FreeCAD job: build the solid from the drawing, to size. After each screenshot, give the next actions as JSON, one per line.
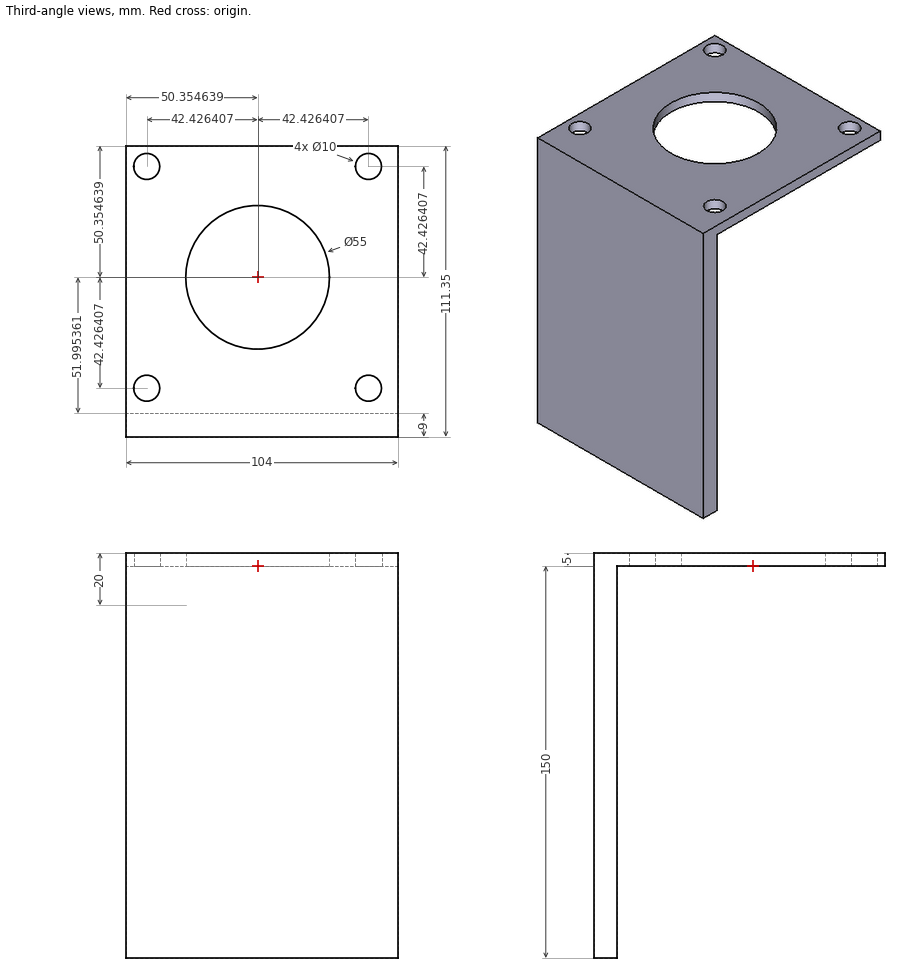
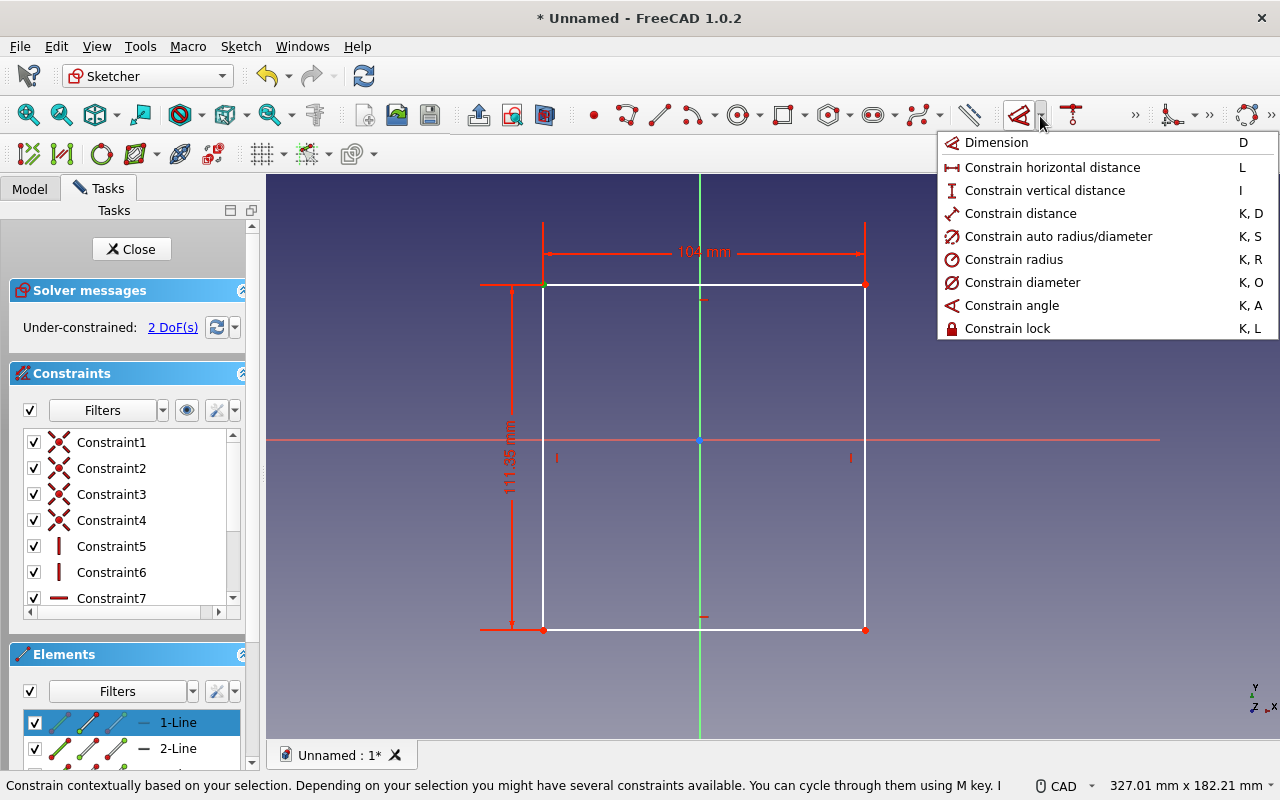
{"action": "left_click", "coordinate": [1108, 168]}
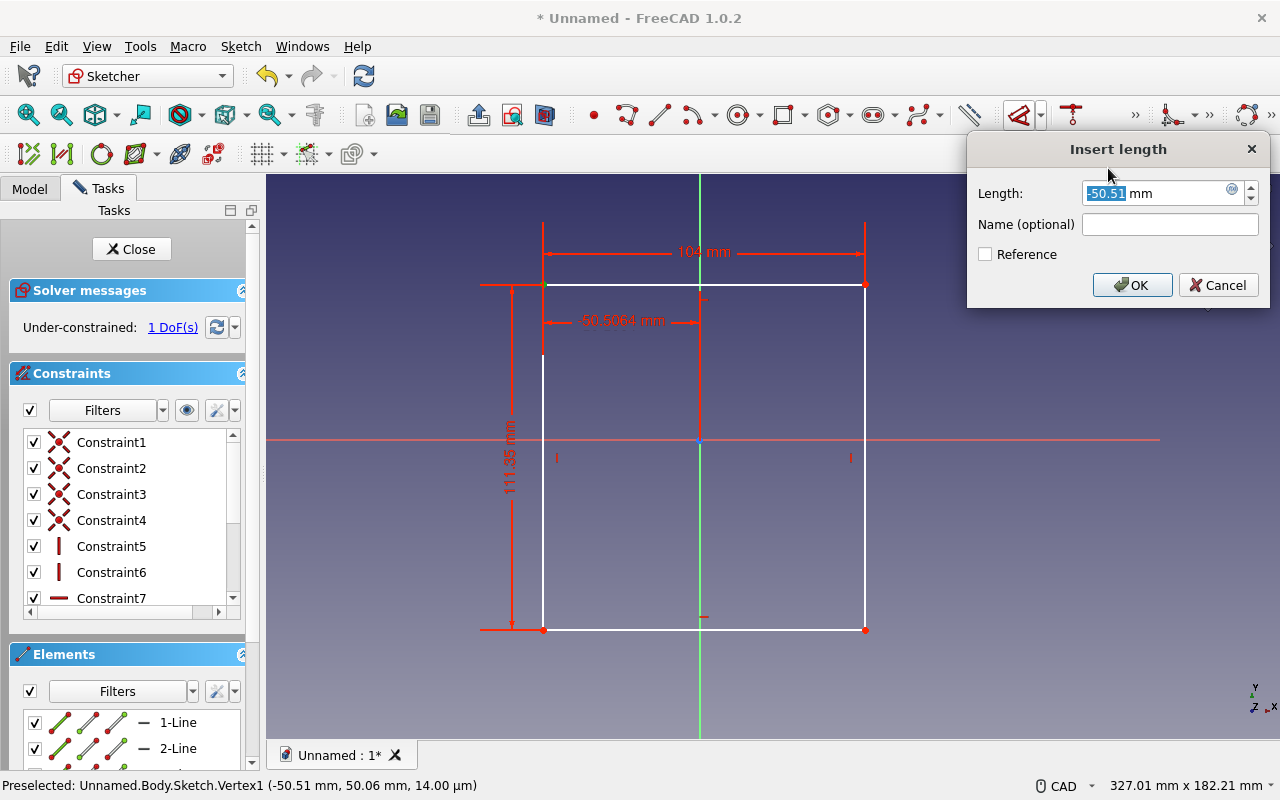
{"action": "type", "text": "-50.354639"}
{"action": "key", "text": "Return"}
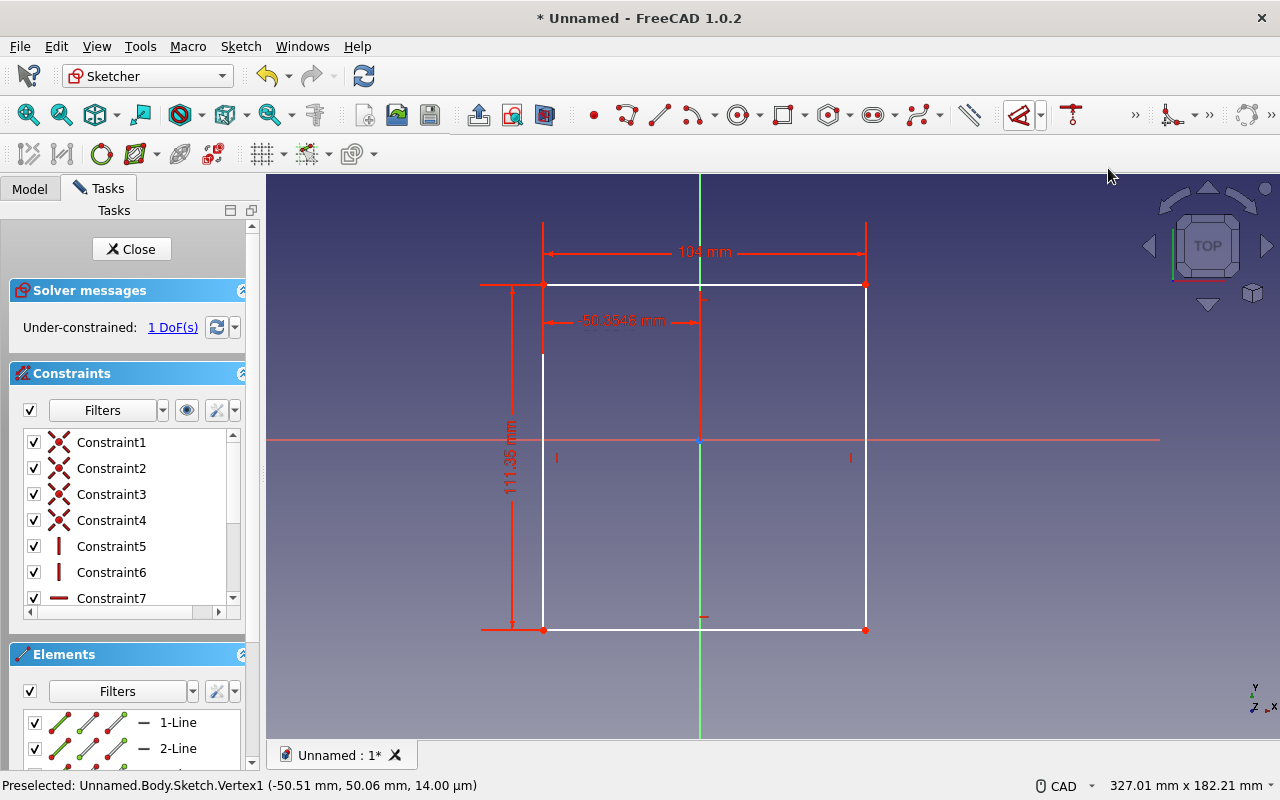
{"action": "left_click", "coordinate": [543, 285]}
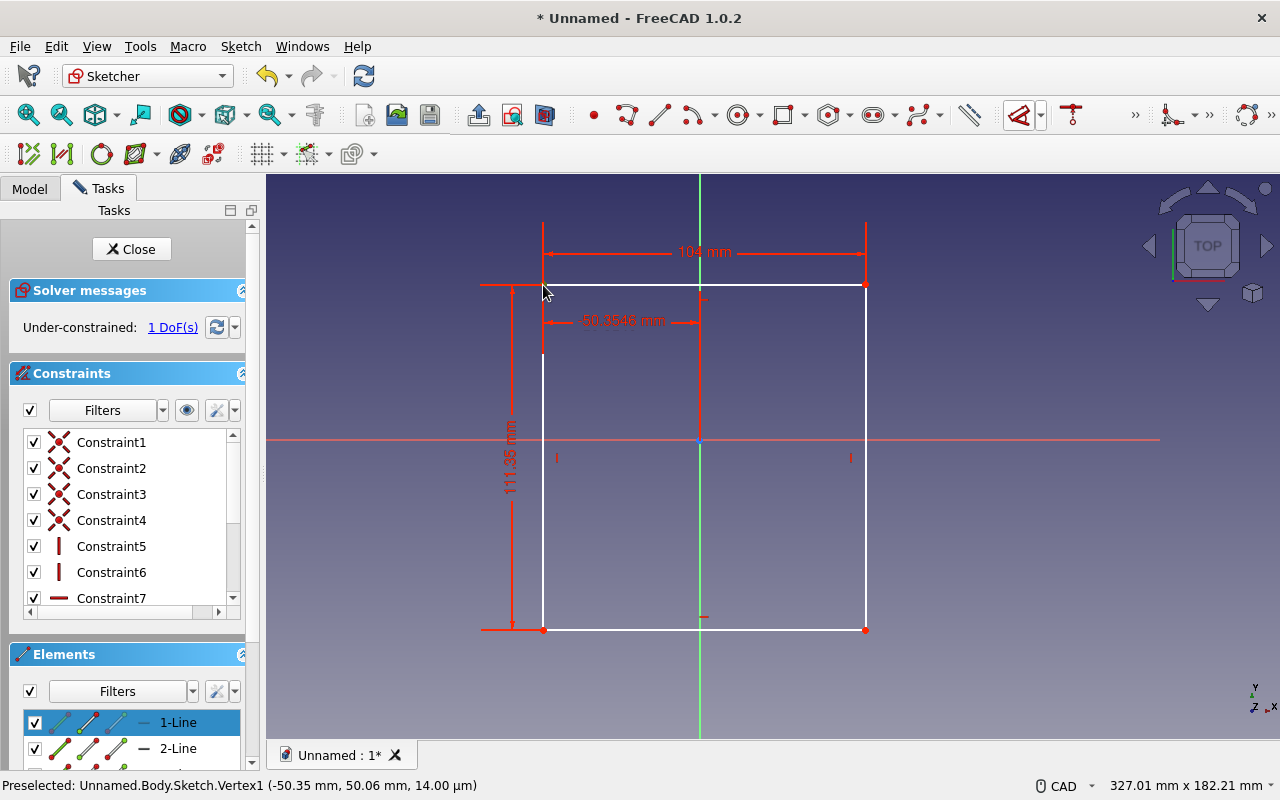
{"action": "key", "text": "i"}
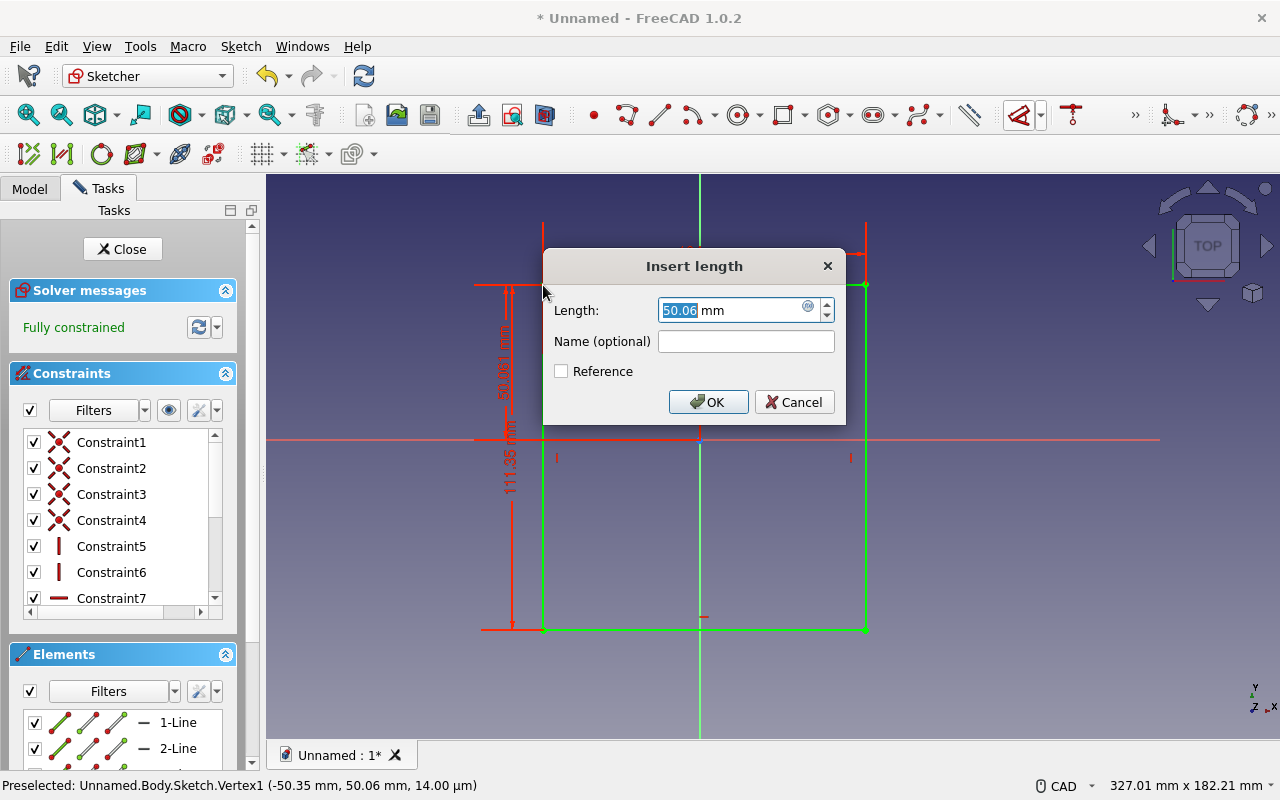
{"action": "type", "text": "50.354639"}
{"action": "key", "text": "Return"}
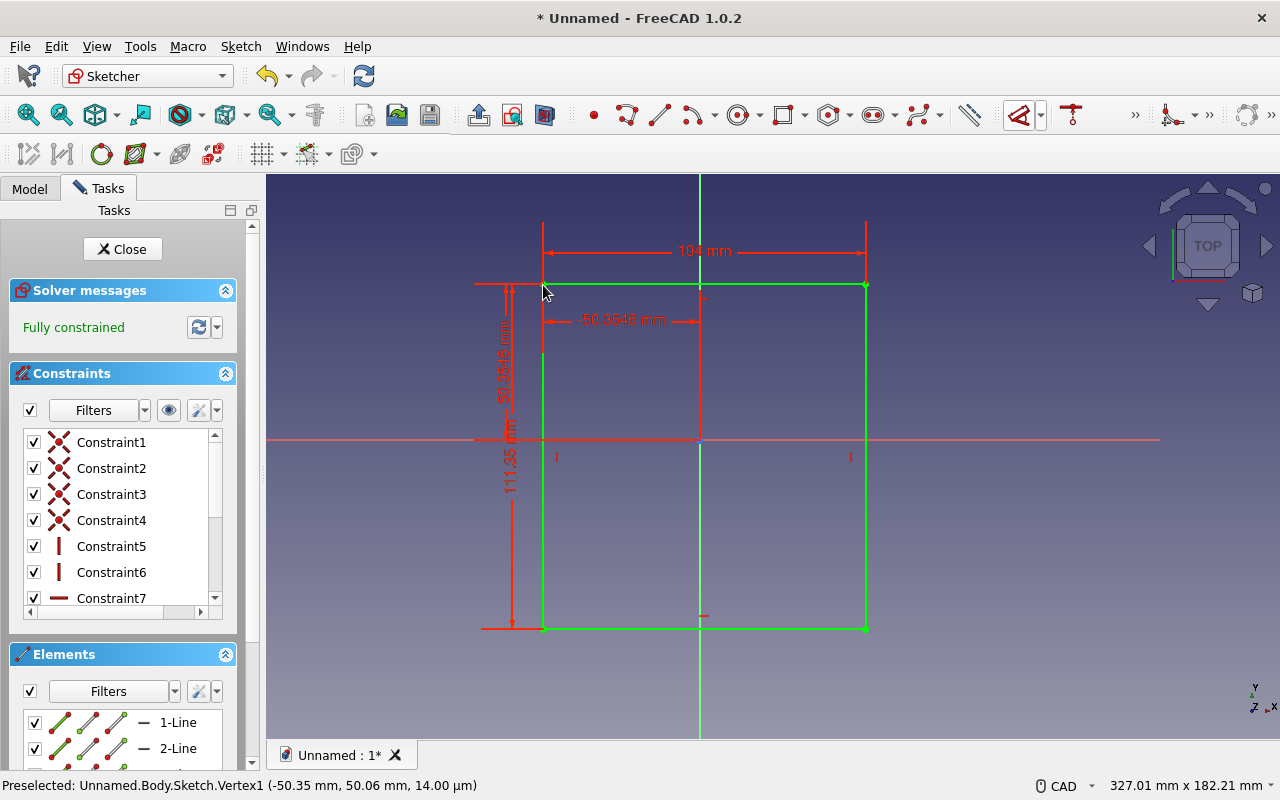
{"action": "left_click", "coordinate": [123, 249]}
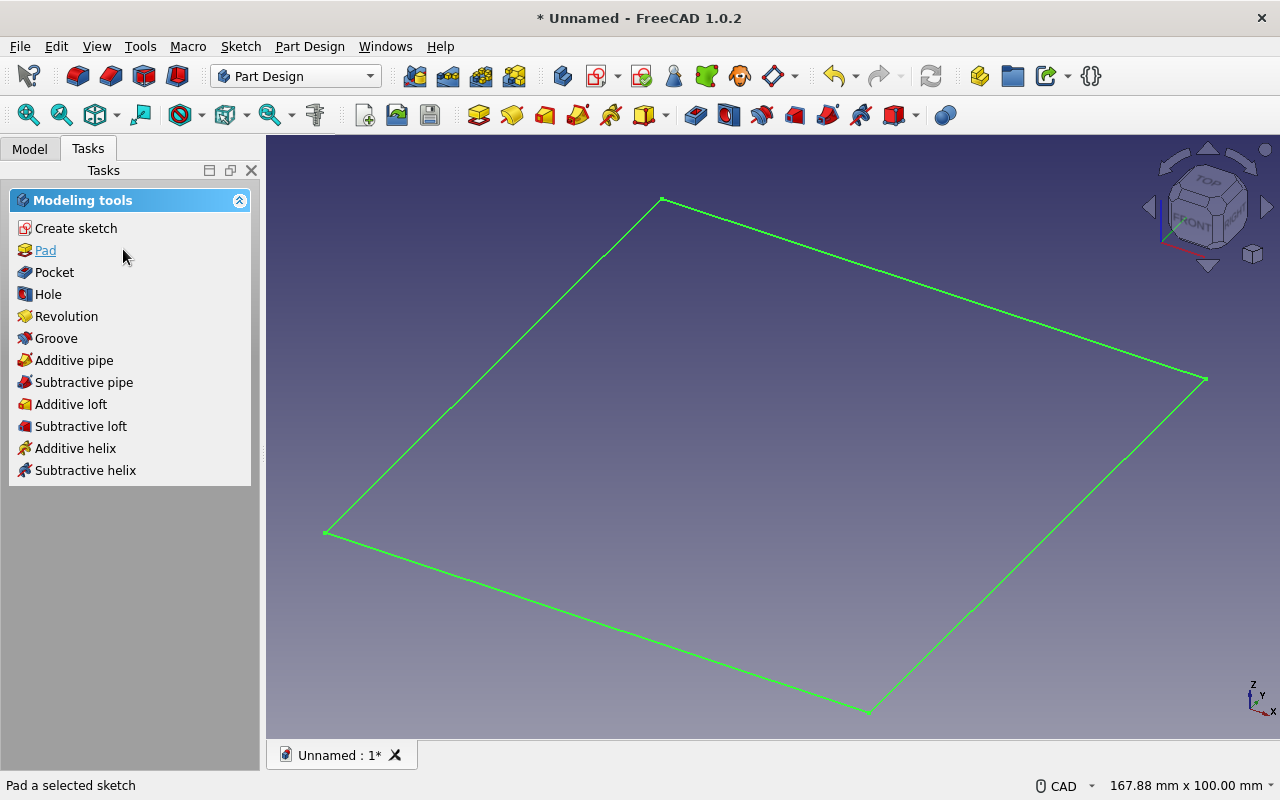
{"action": "left_click", "coordinate": [479, 116]}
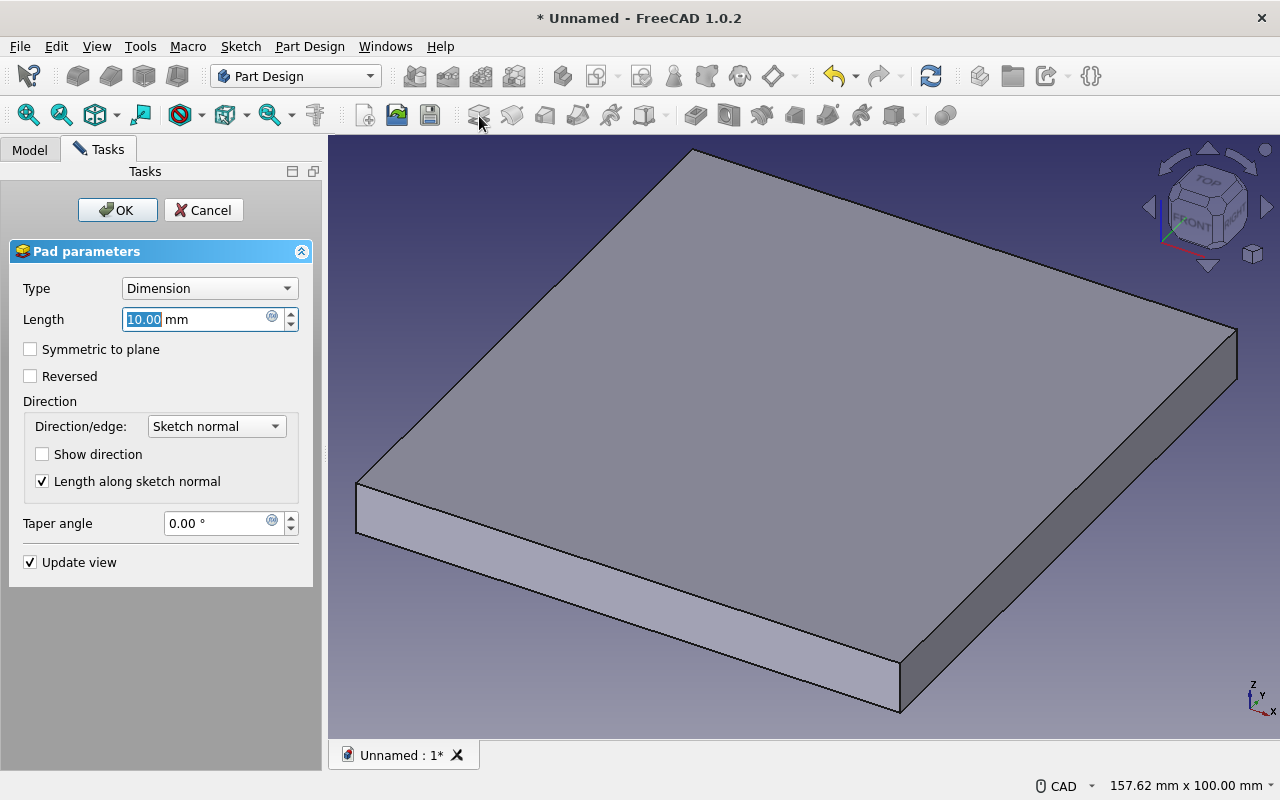
{"action": "type", "text": "5"}
{"action": "key", "text": "Tab"}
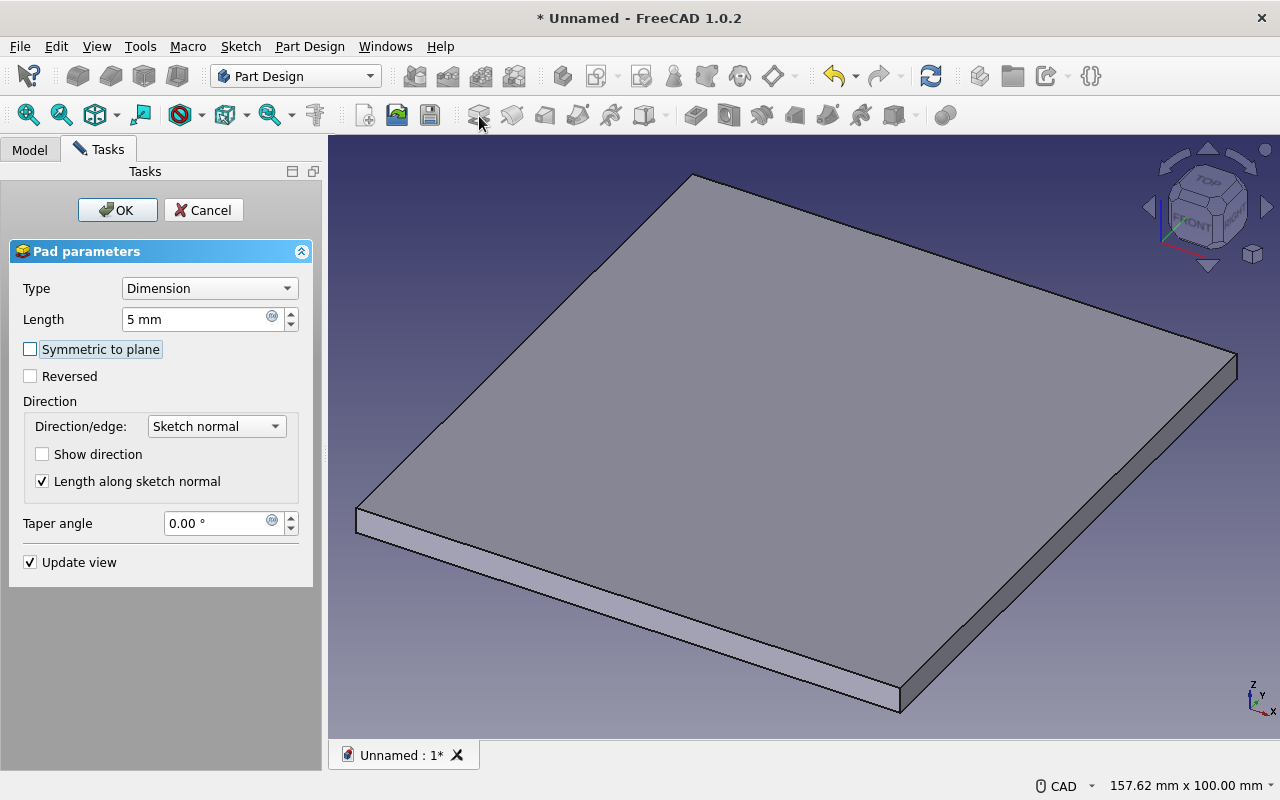
{"action": "left_click", "coordinate": [118, 210]}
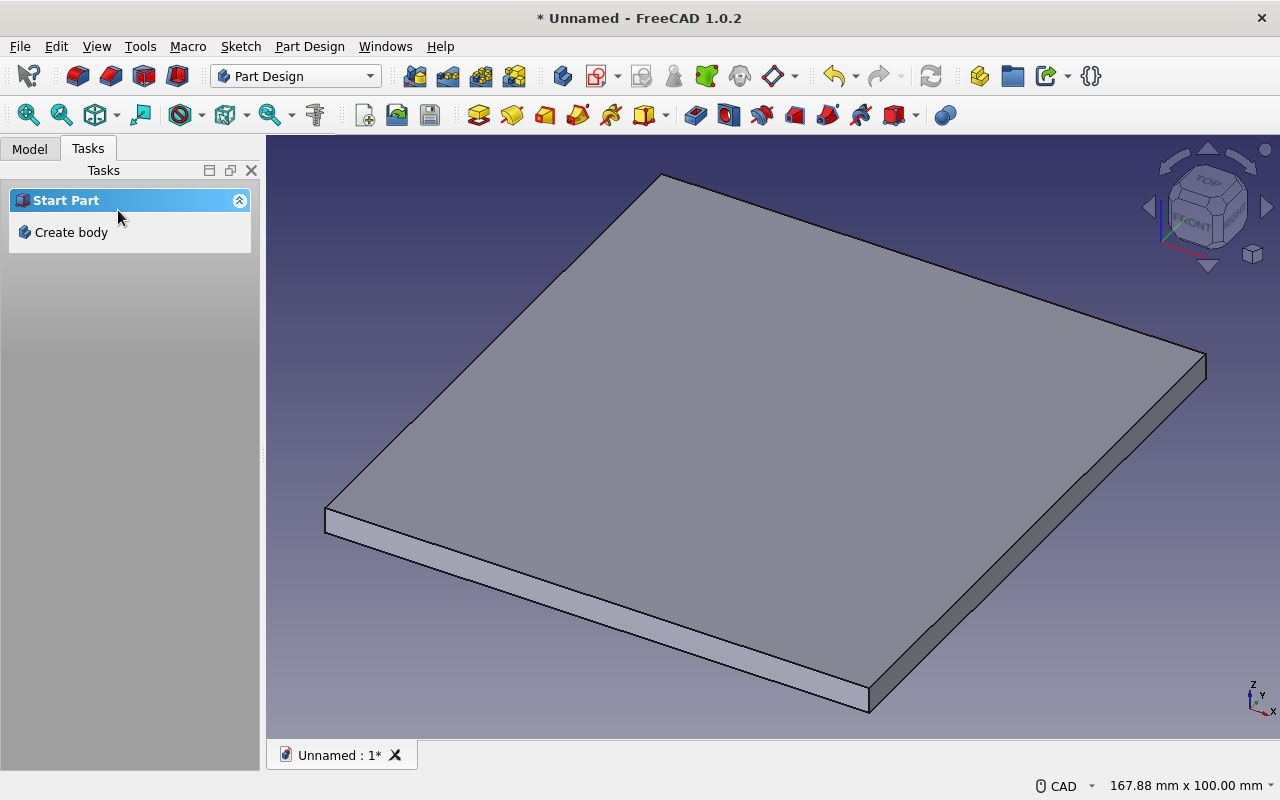
{"action": "left_click", "coordinate": [766, 430]}